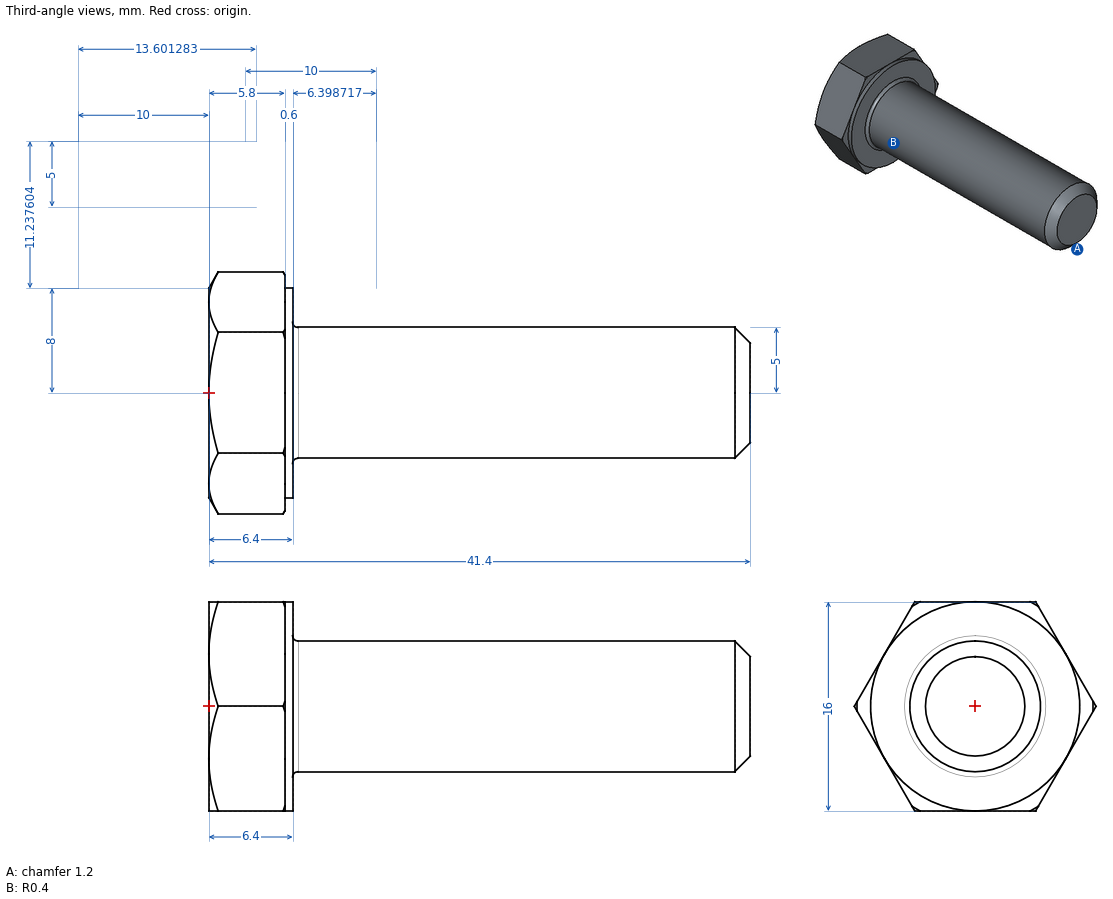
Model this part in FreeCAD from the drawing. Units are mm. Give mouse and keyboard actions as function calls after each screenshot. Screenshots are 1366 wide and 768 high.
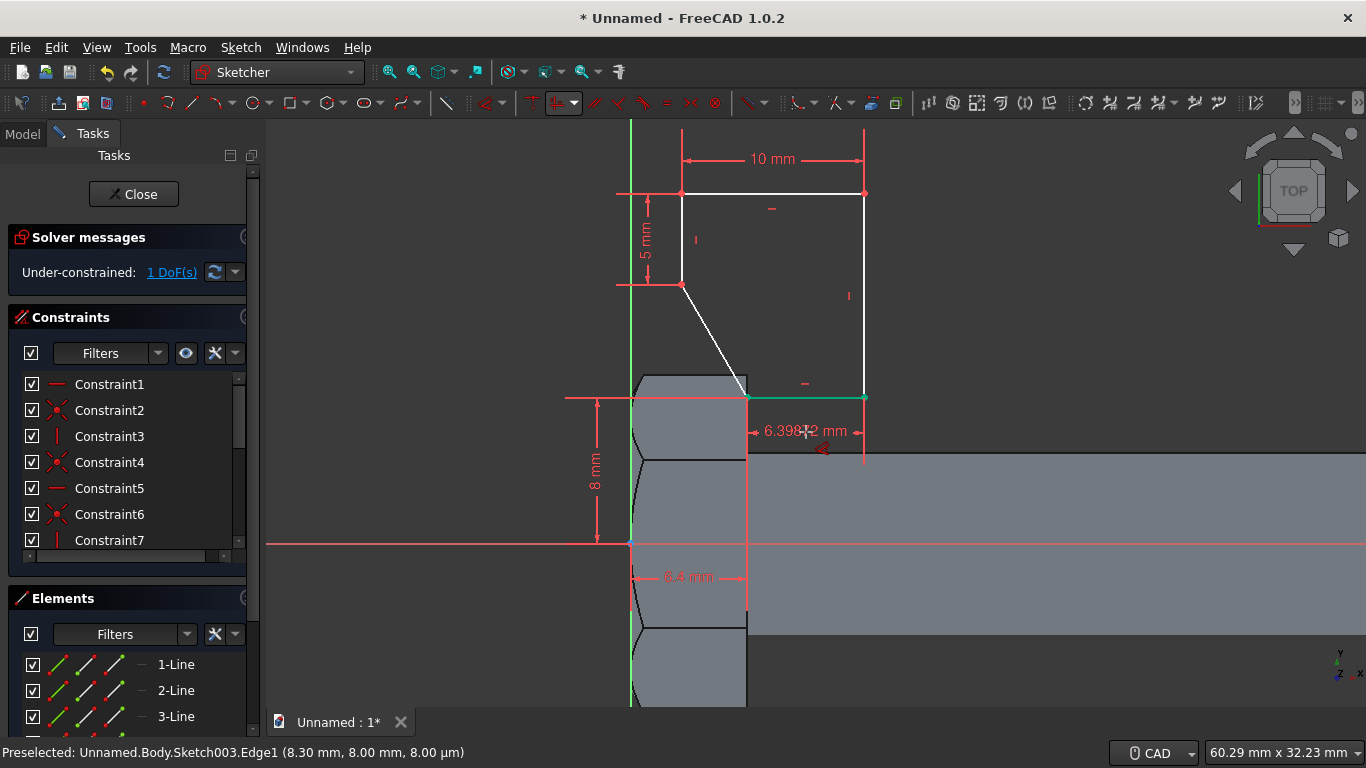
click(864, 337)
click(898, 296)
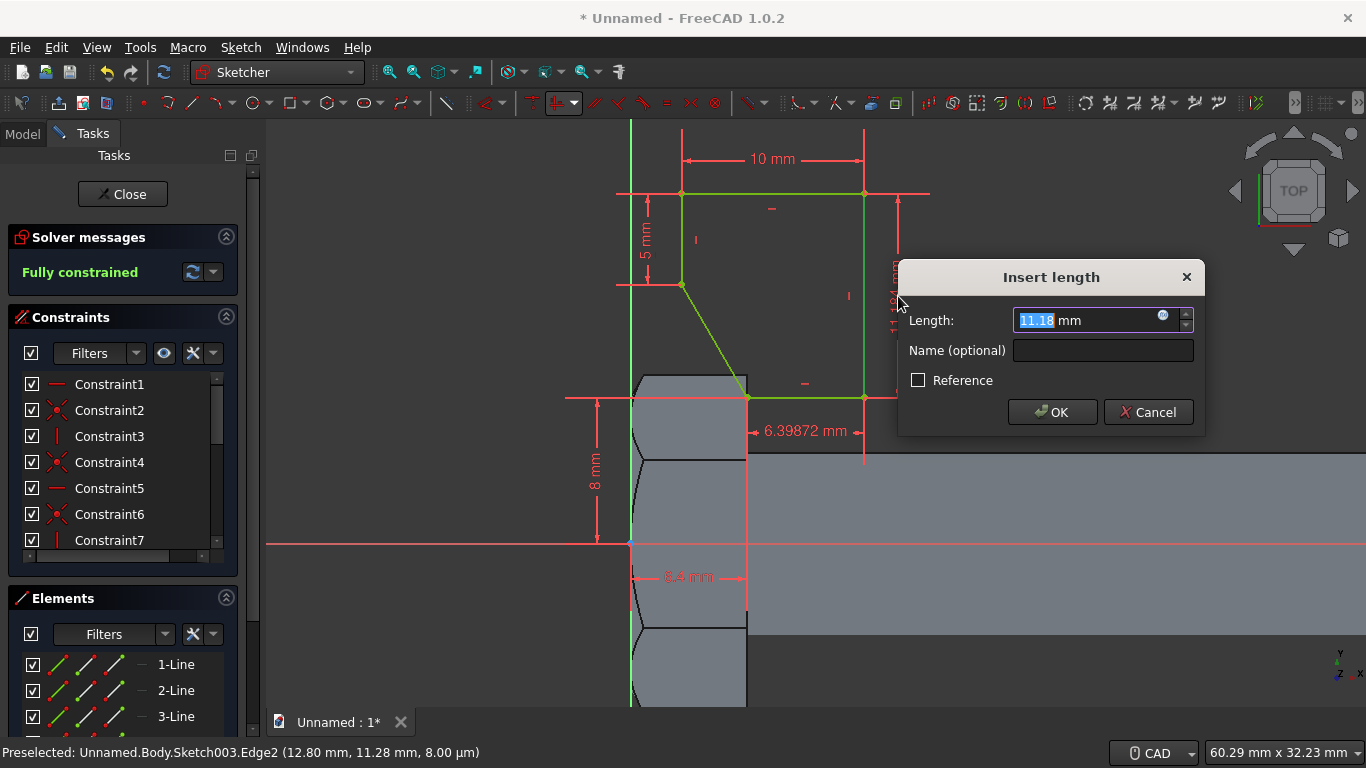
text(11.237604)
key(Return)
key(Escape)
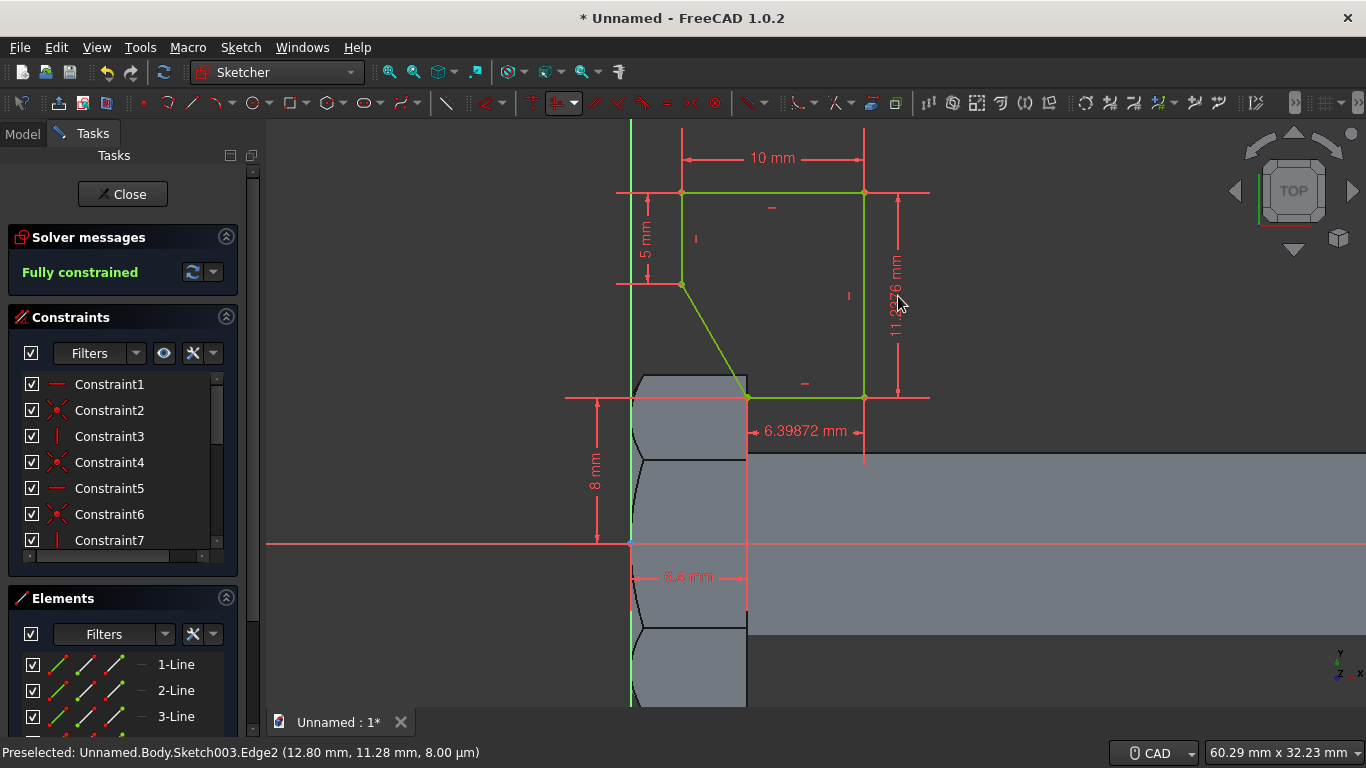
click(123, 194)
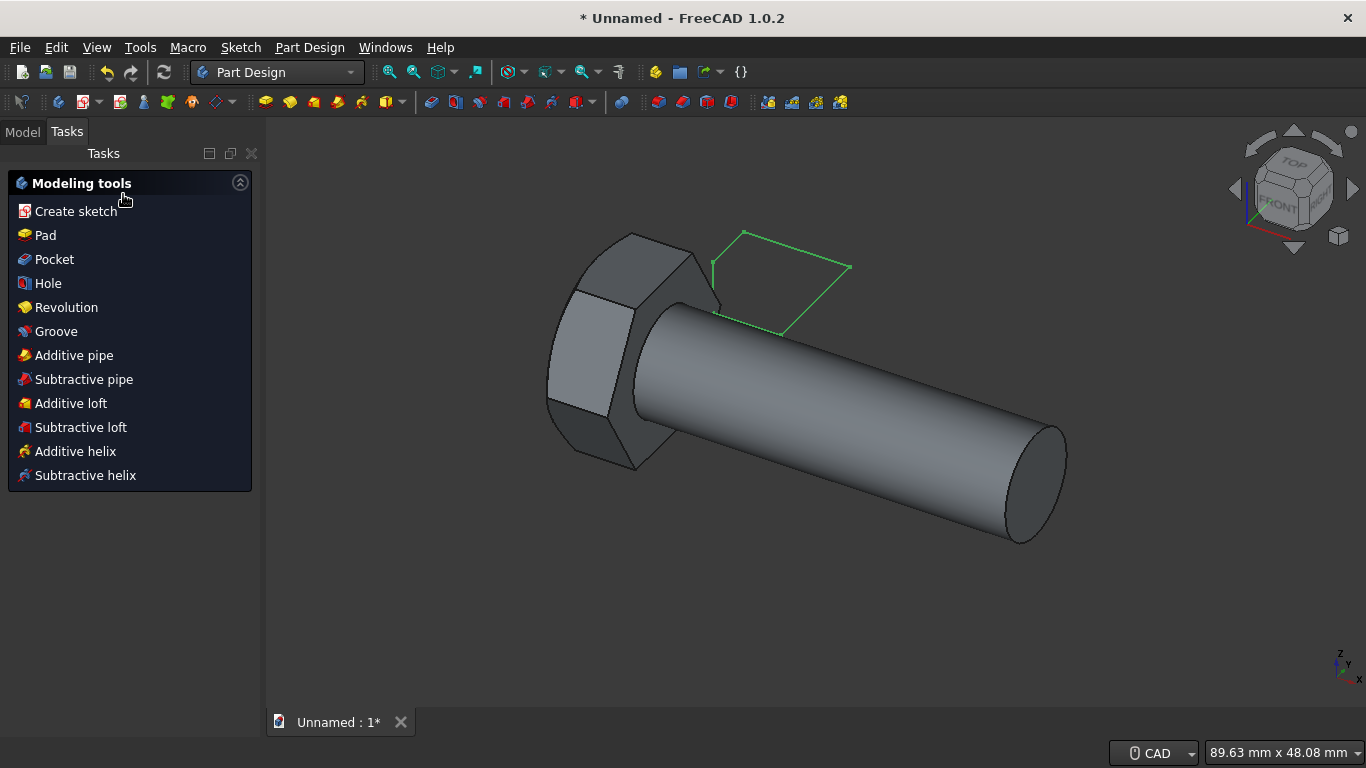
click(480, 102)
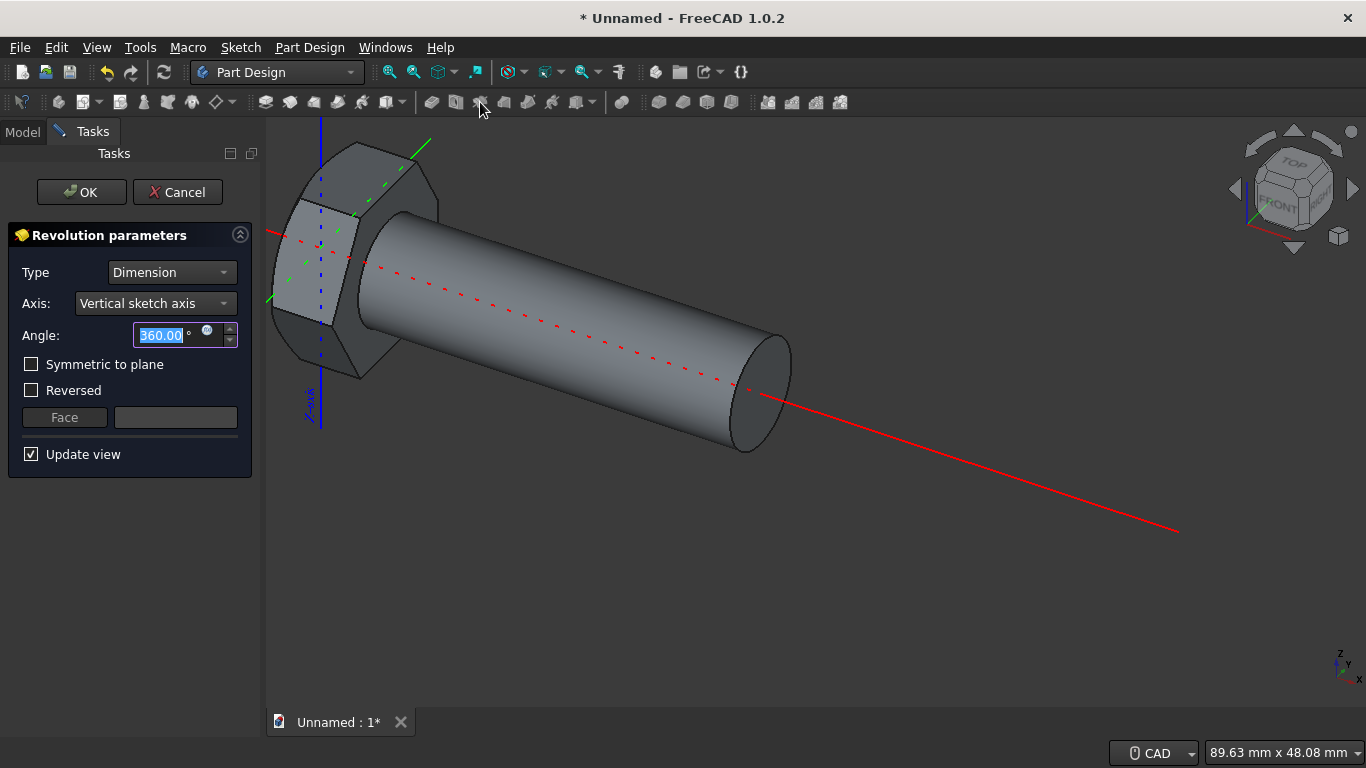
click(156, 304)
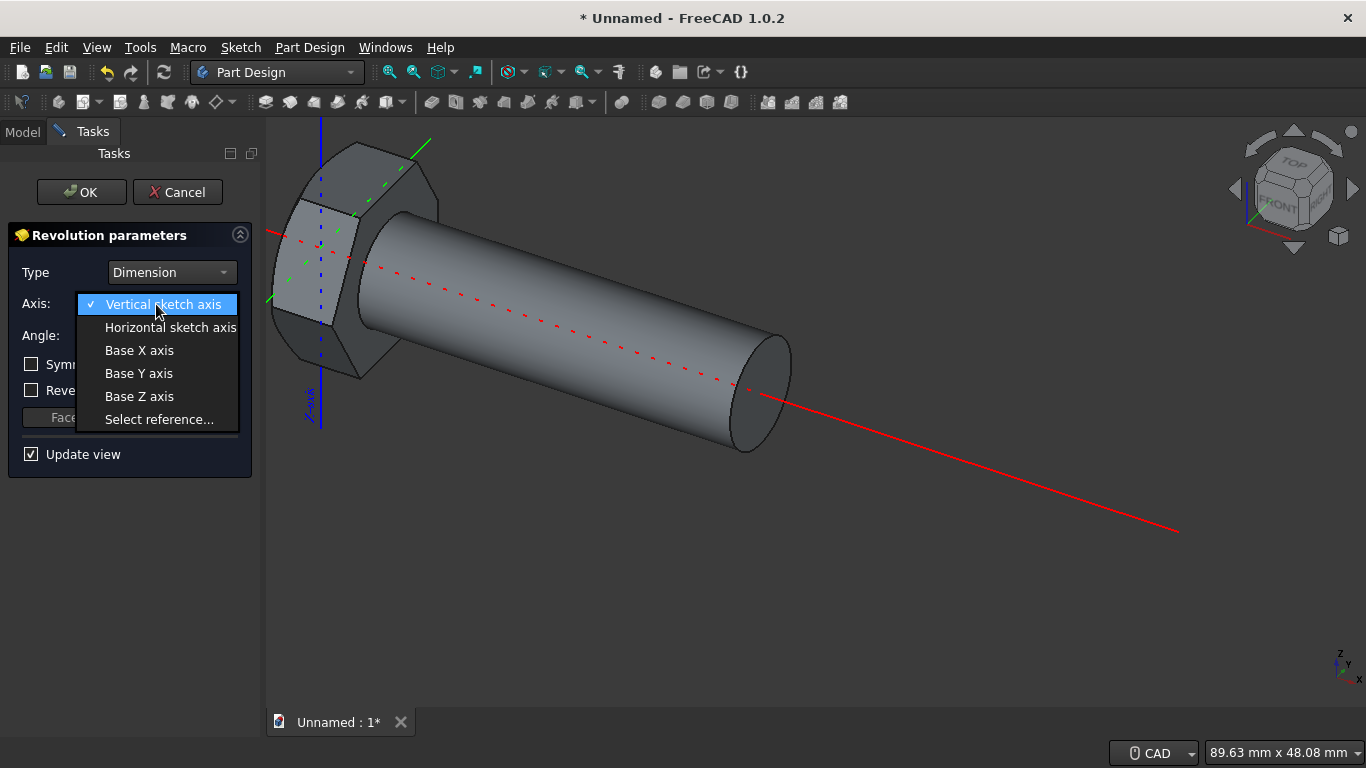
click(156, 328)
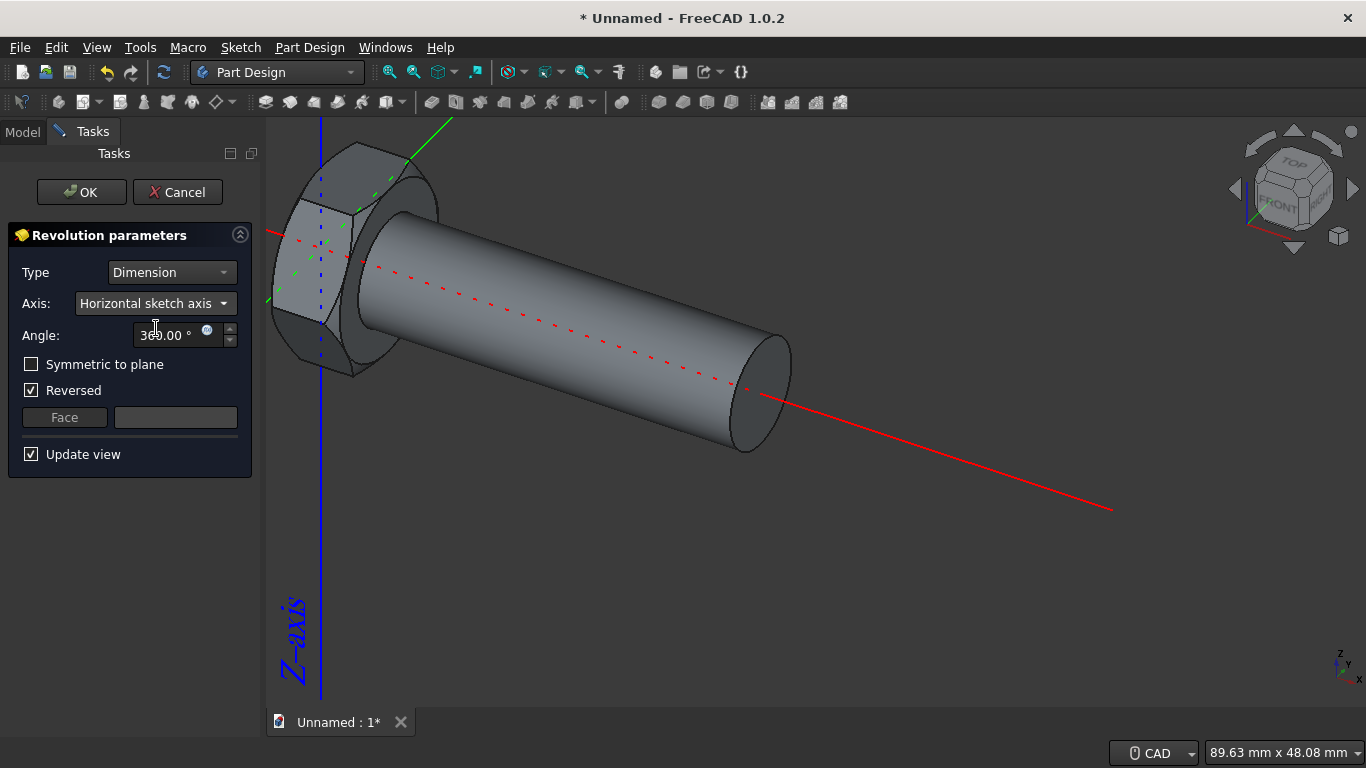
click(82, 192)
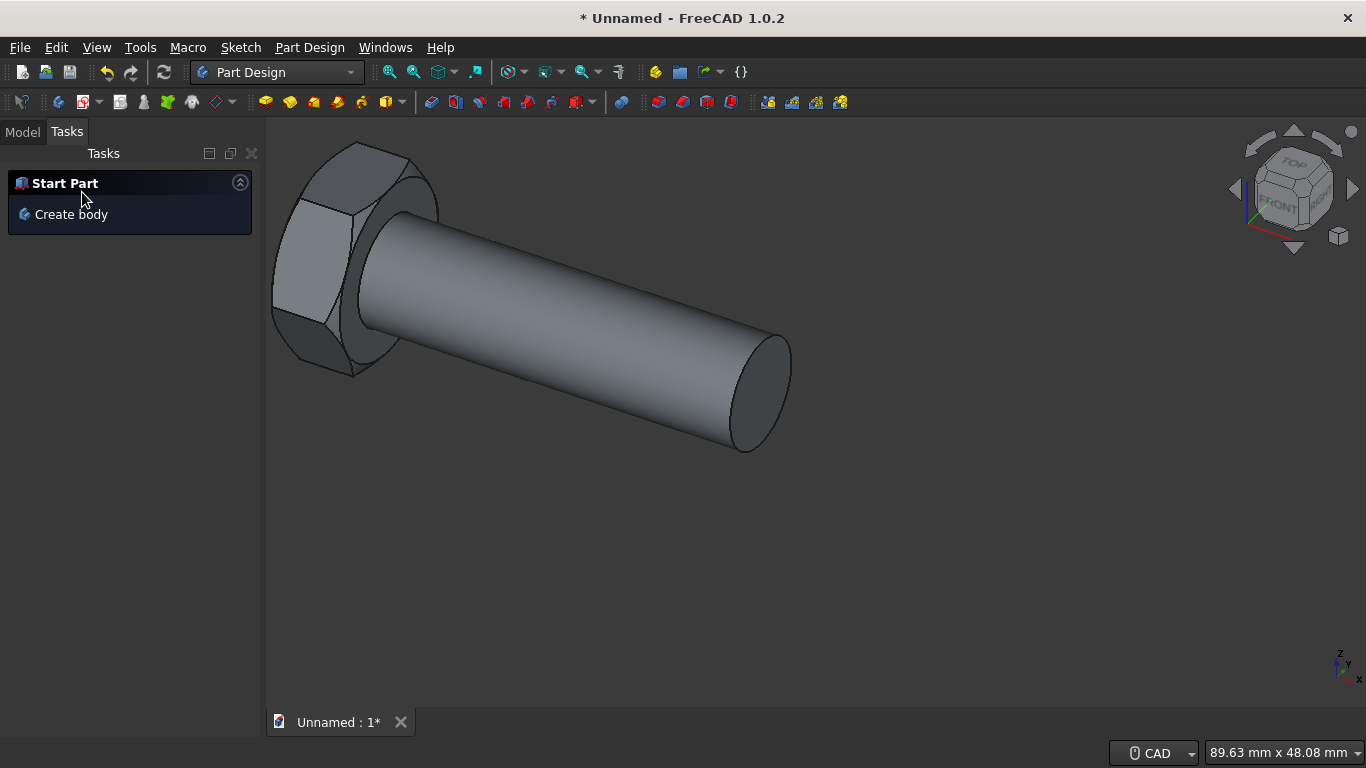
key(v)
key(f)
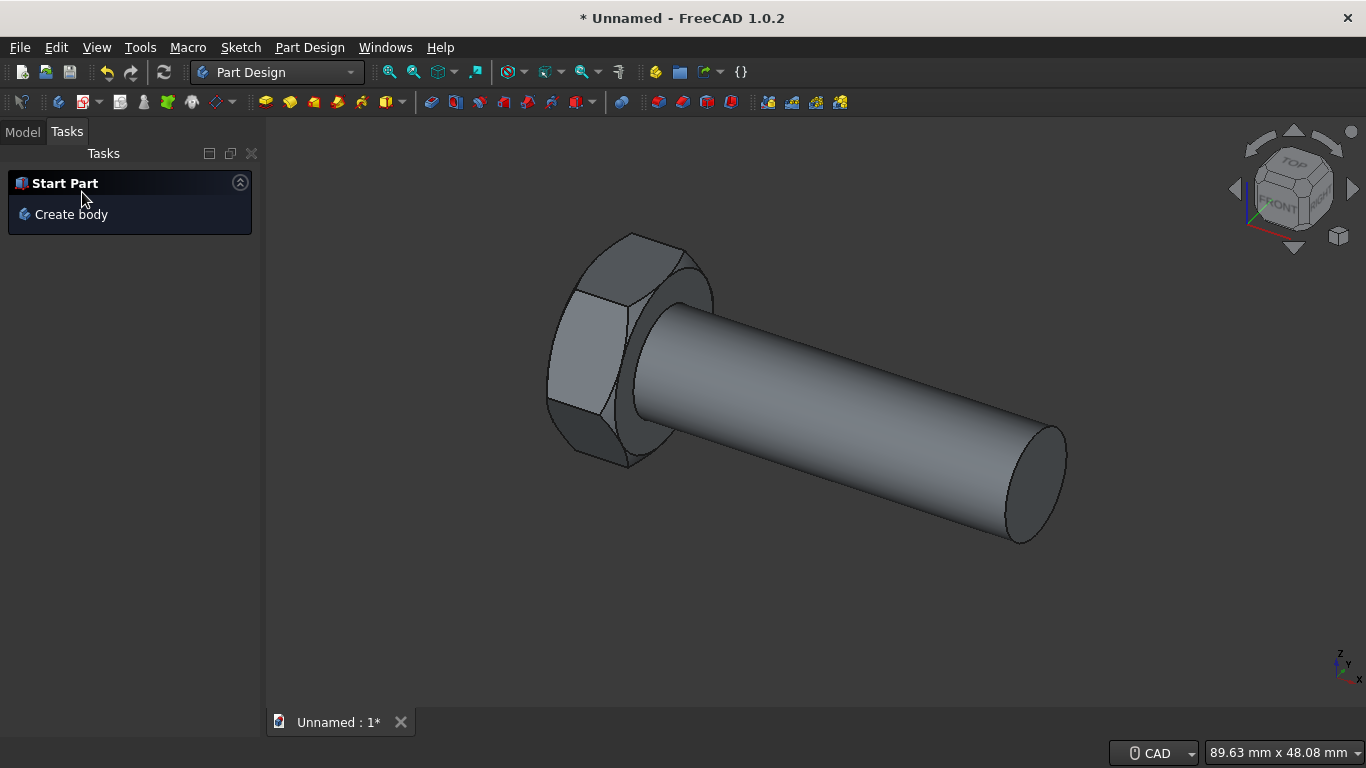
click(84, 102)